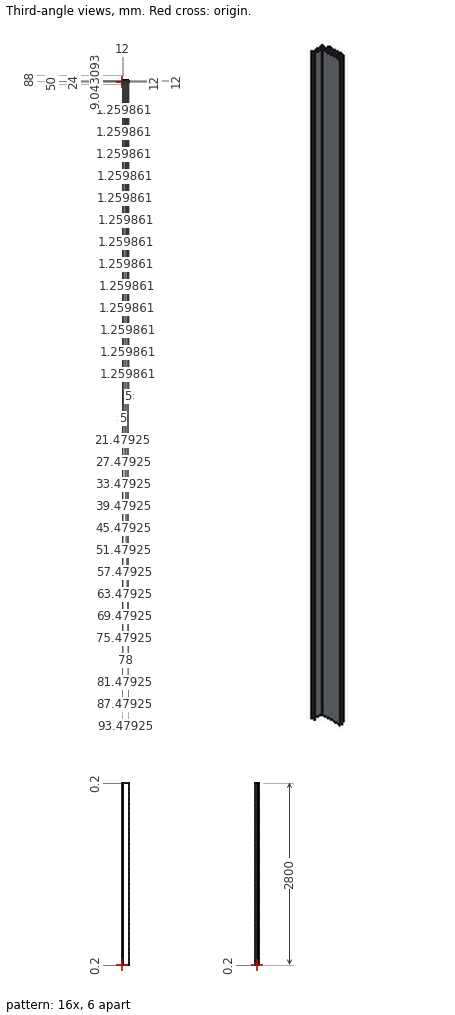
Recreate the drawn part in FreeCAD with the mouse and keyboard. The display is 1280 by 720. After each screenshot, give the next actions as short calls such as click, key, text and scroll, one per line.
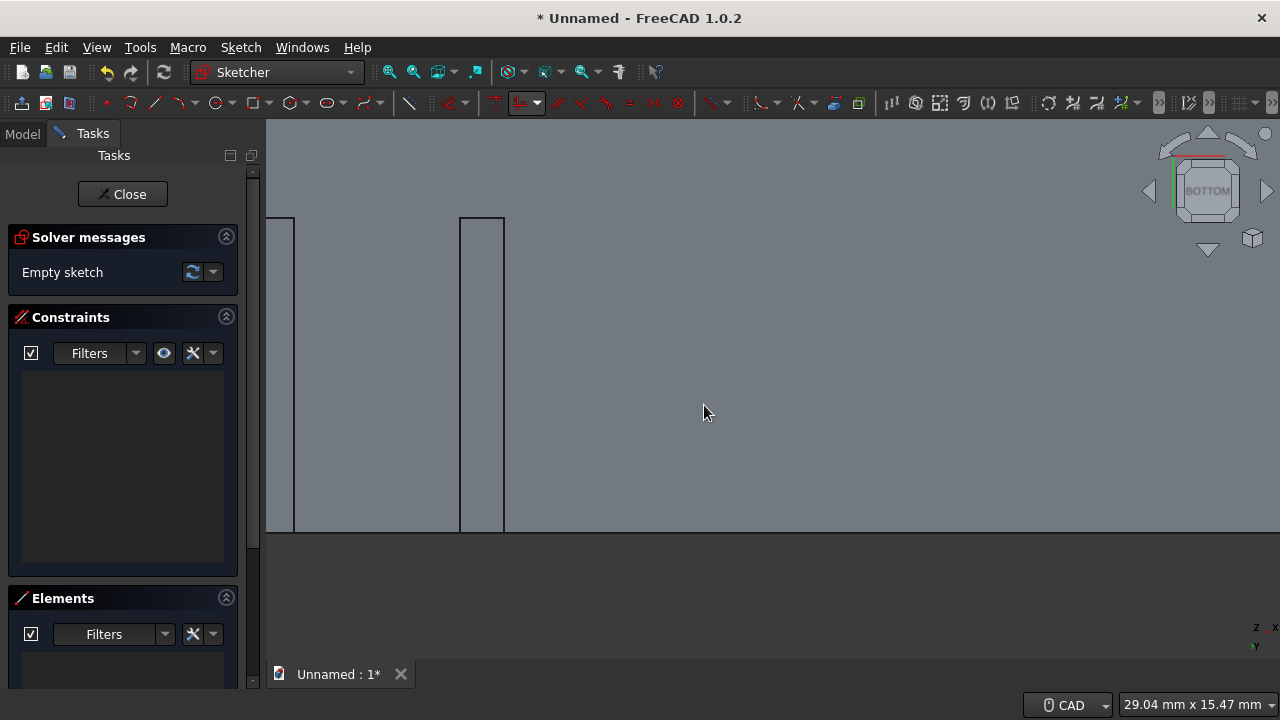
click(254, 104)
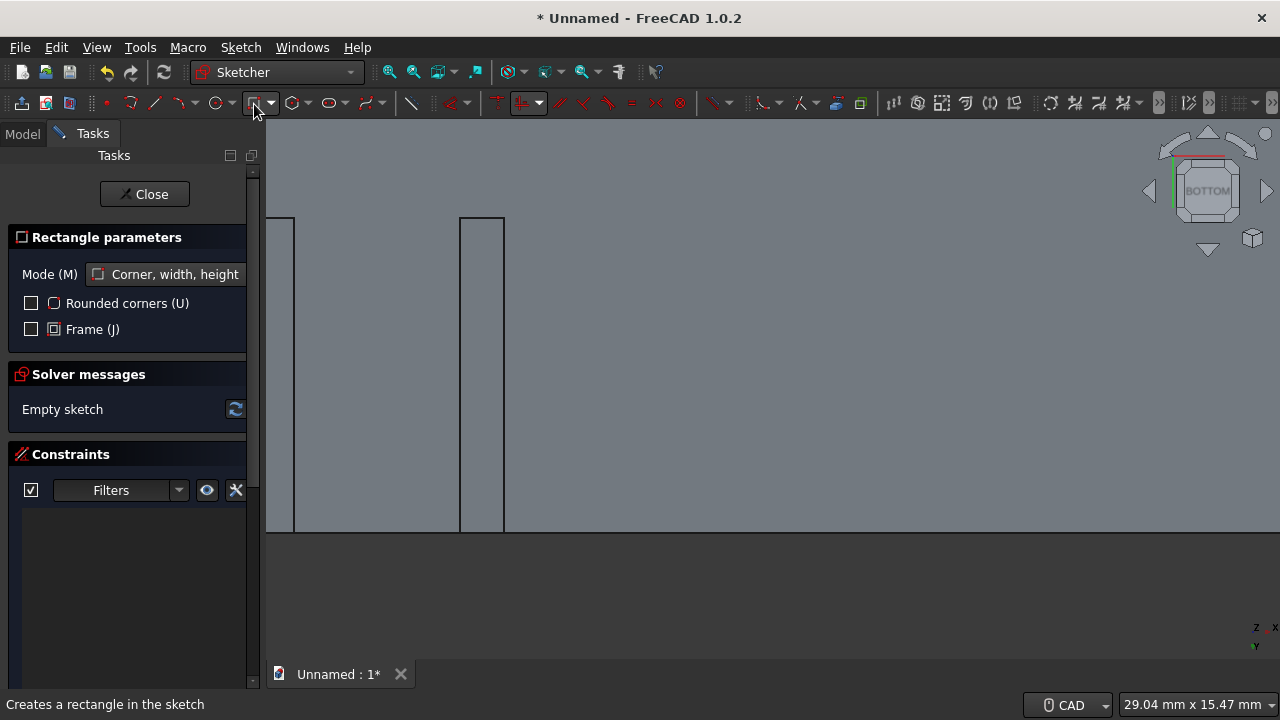
click(669, 218)
move(713, 533)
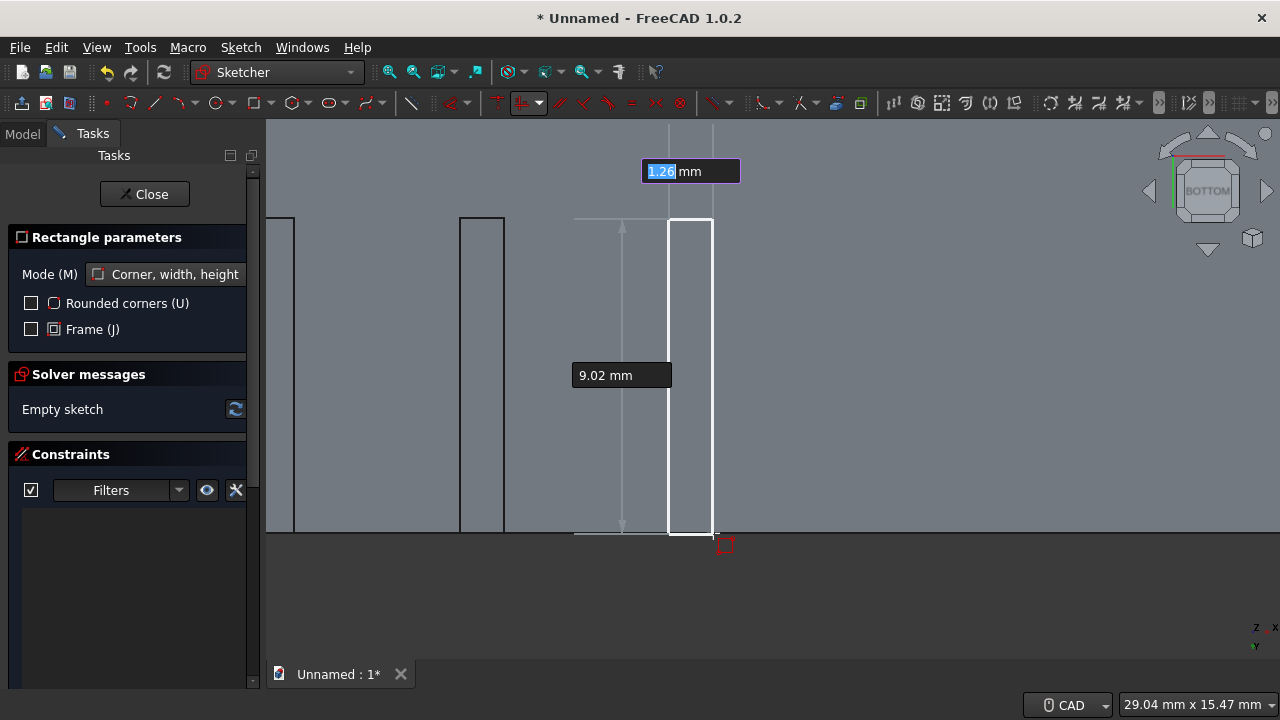
text(1.259861)
key(Tab)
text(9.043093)
key(Return)
key(Escape)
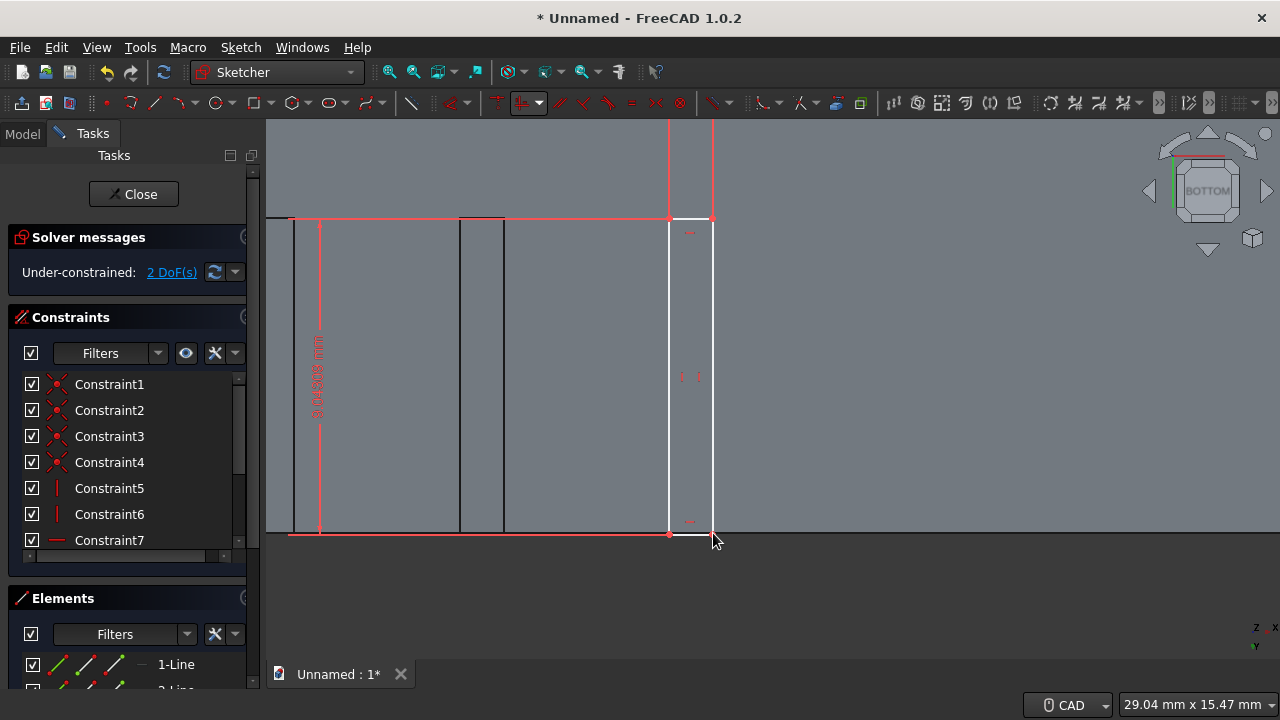
click(450, 104)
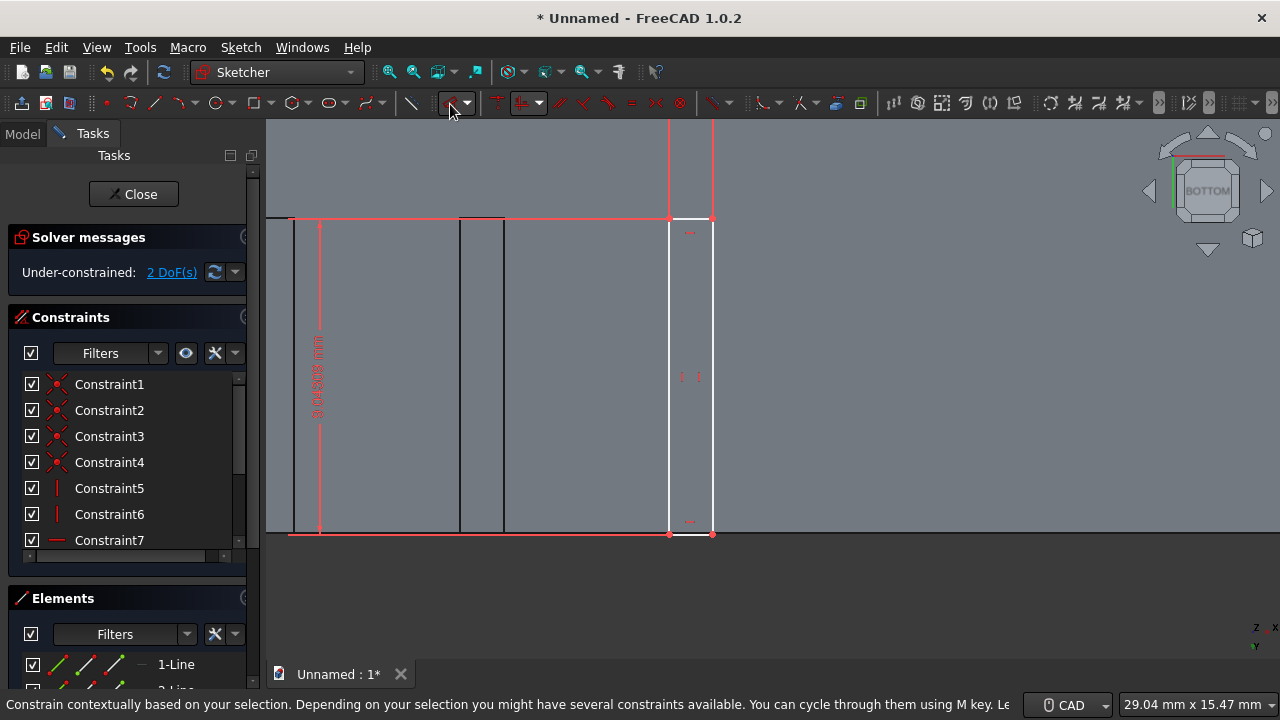
click(669, 535)
click(703, 205)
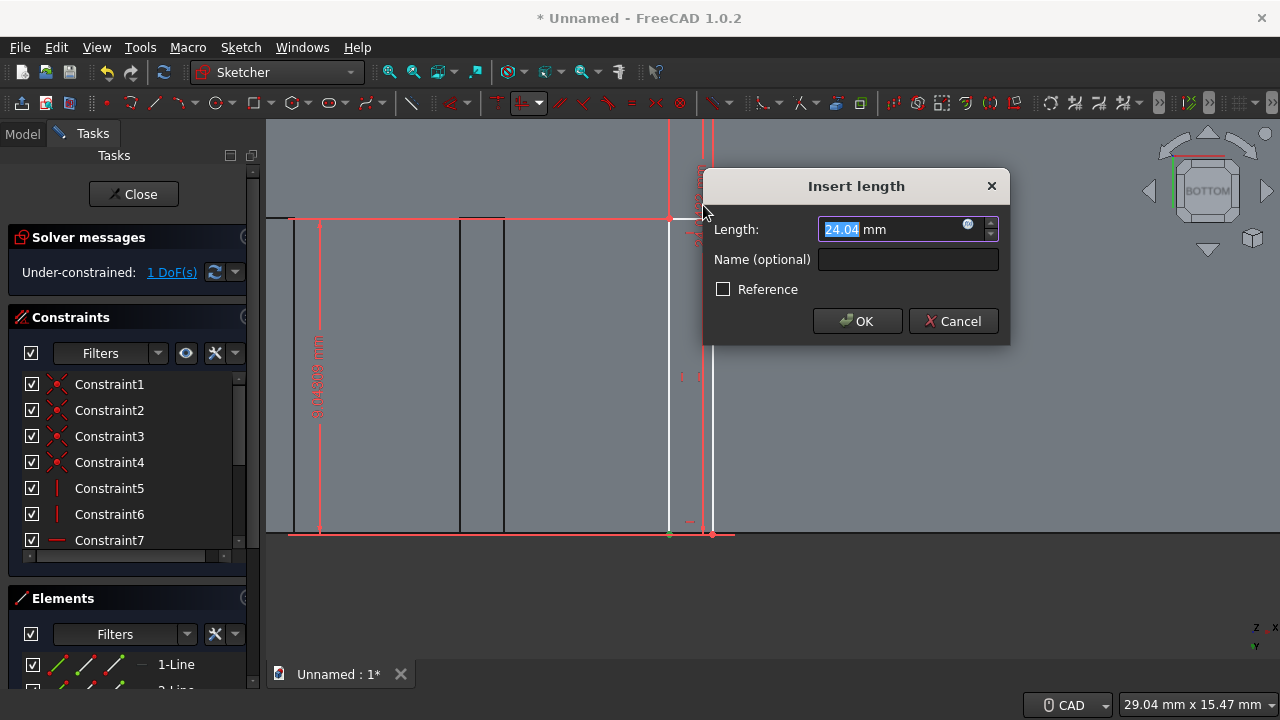
text(24)
key(Return)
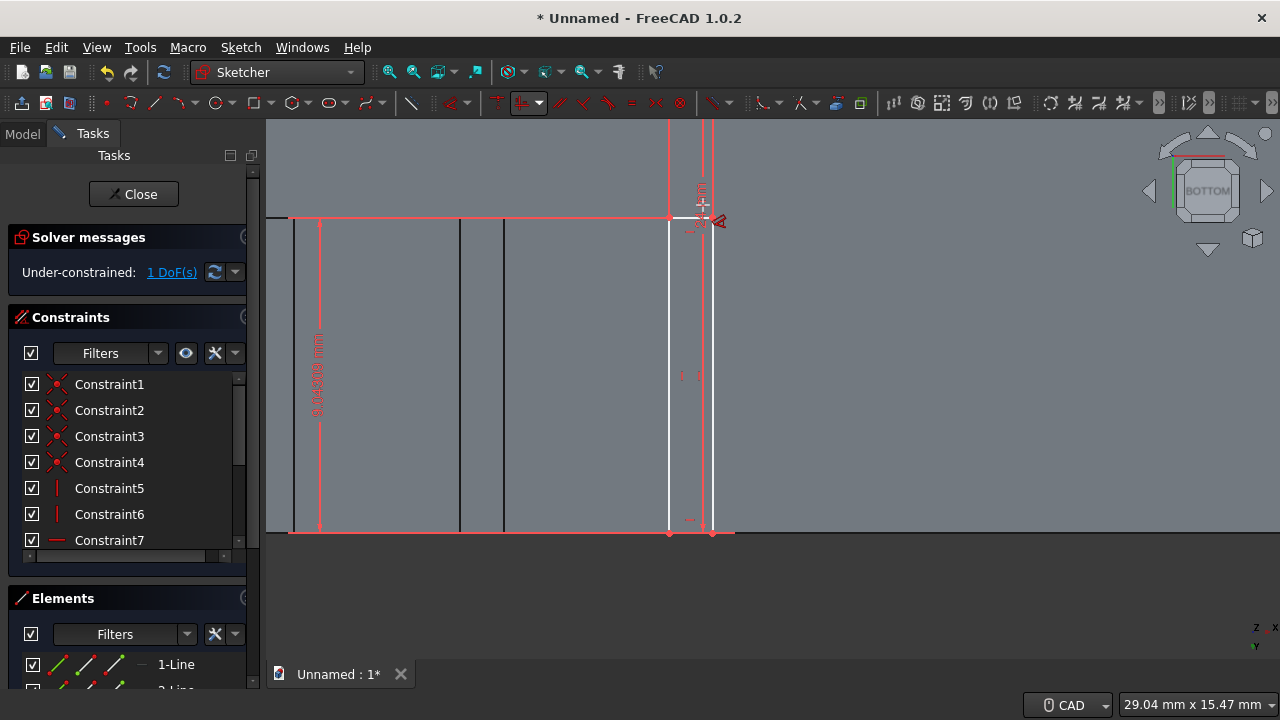
click(669, 218)
click(481, 252)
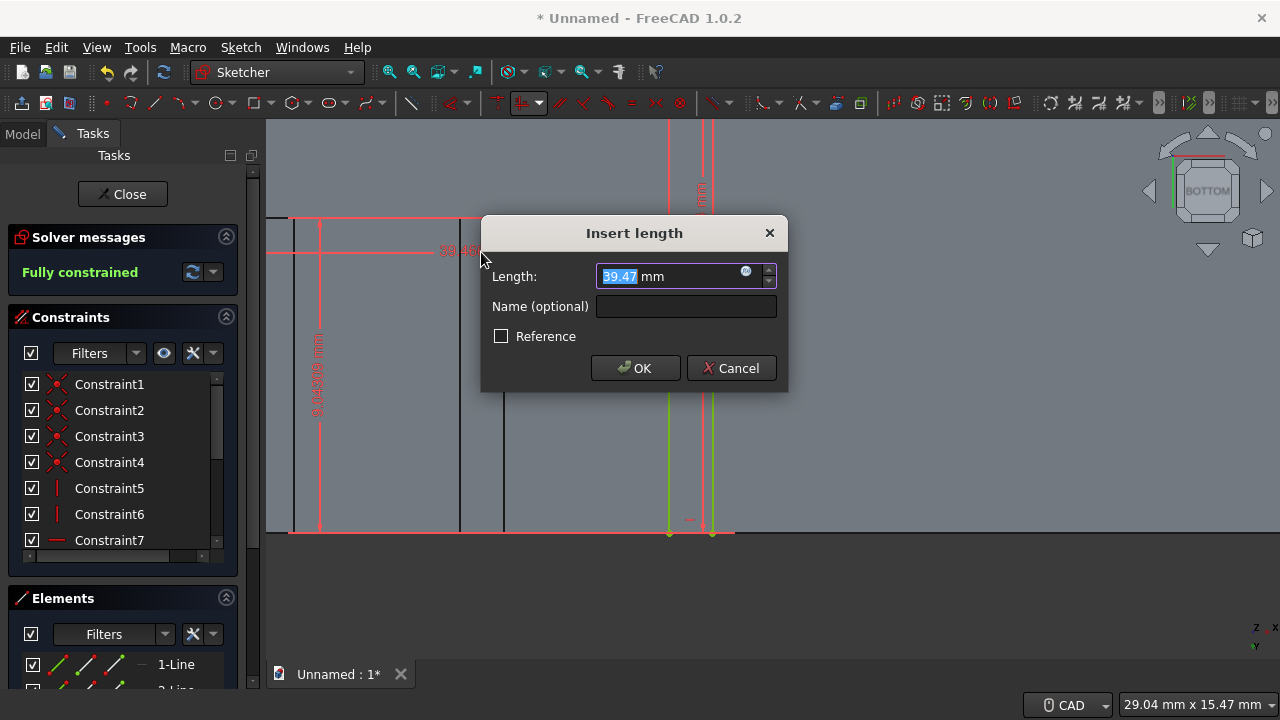
text(39.47925)
key(Return)
key(Escape)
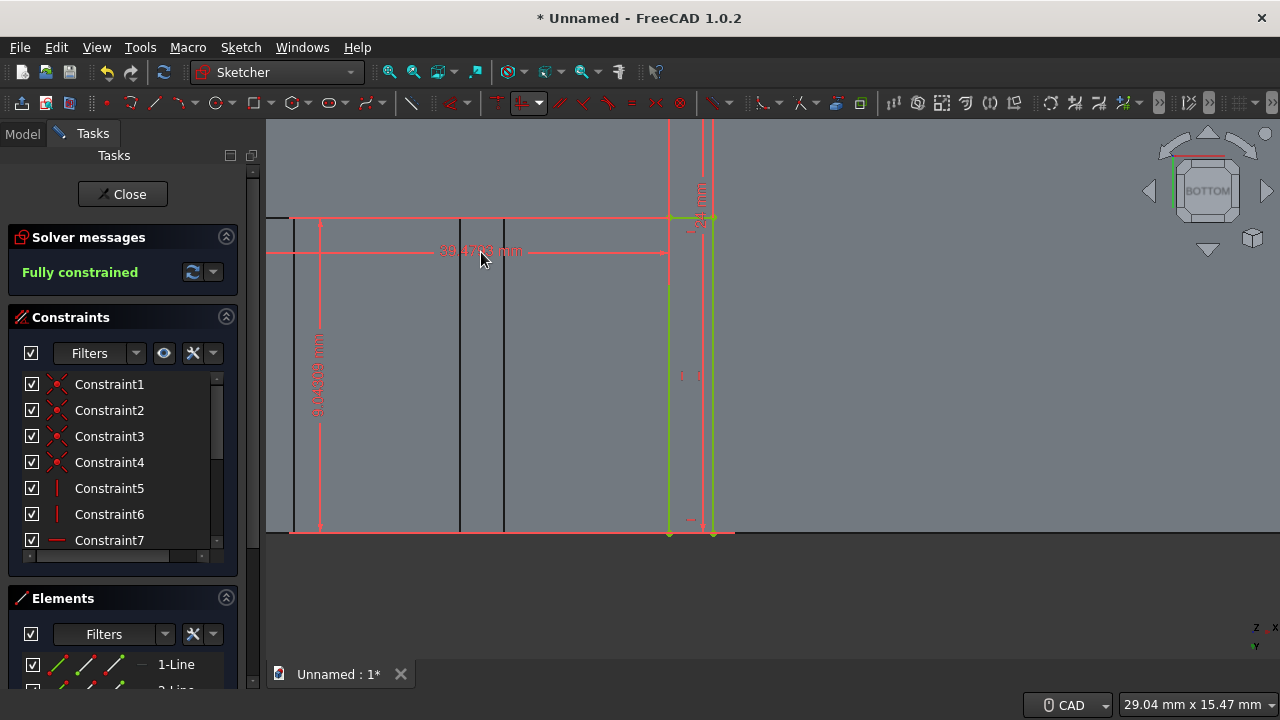
click(123, 194)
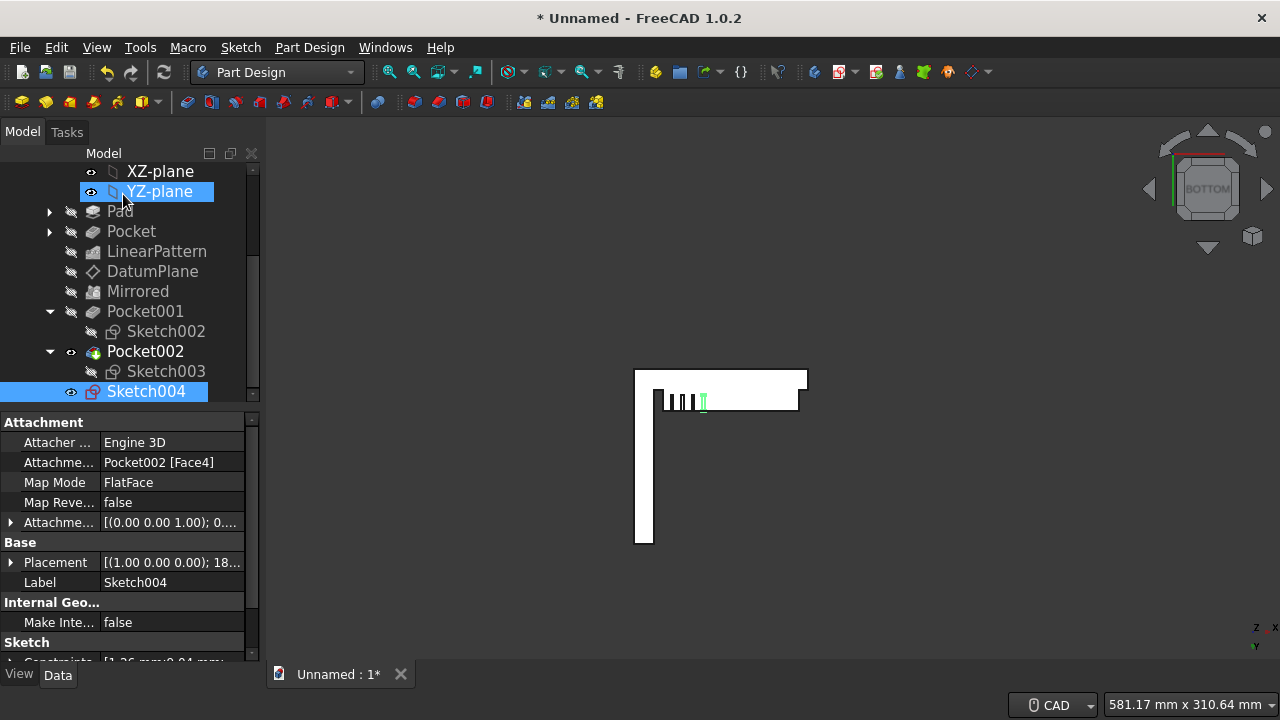
click(188, 102)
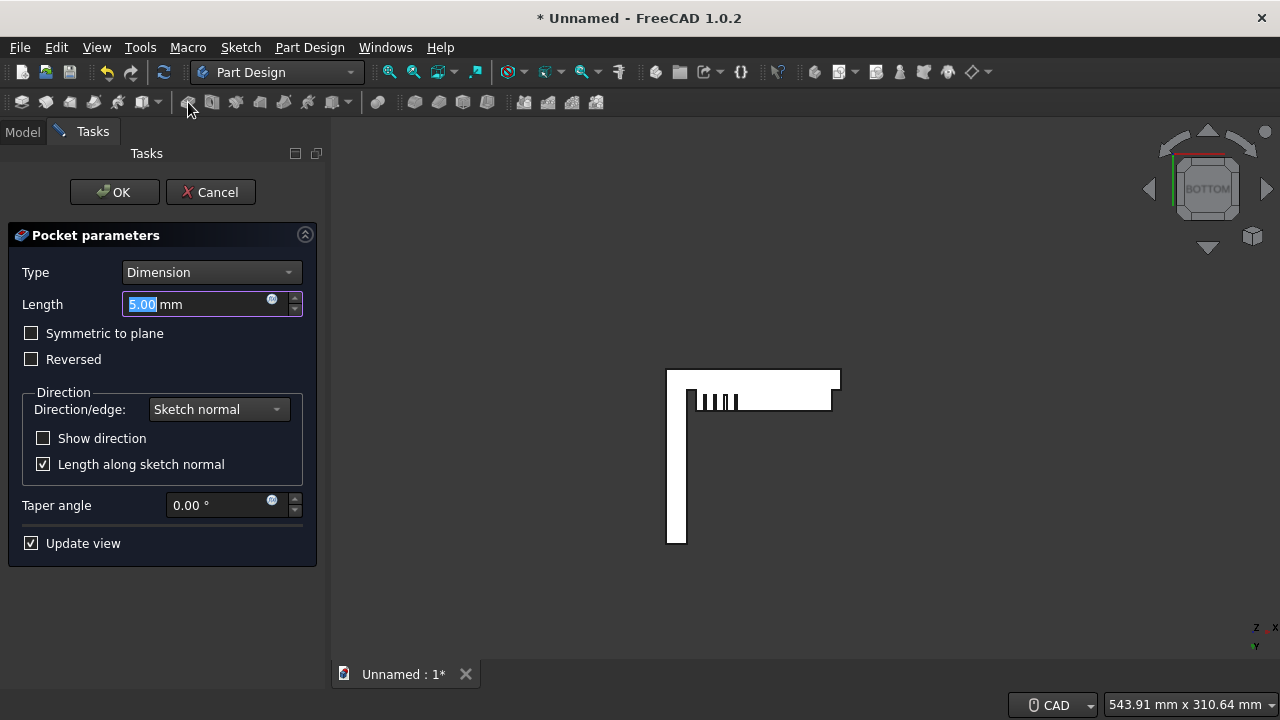
text(0.2)
key(Tab)